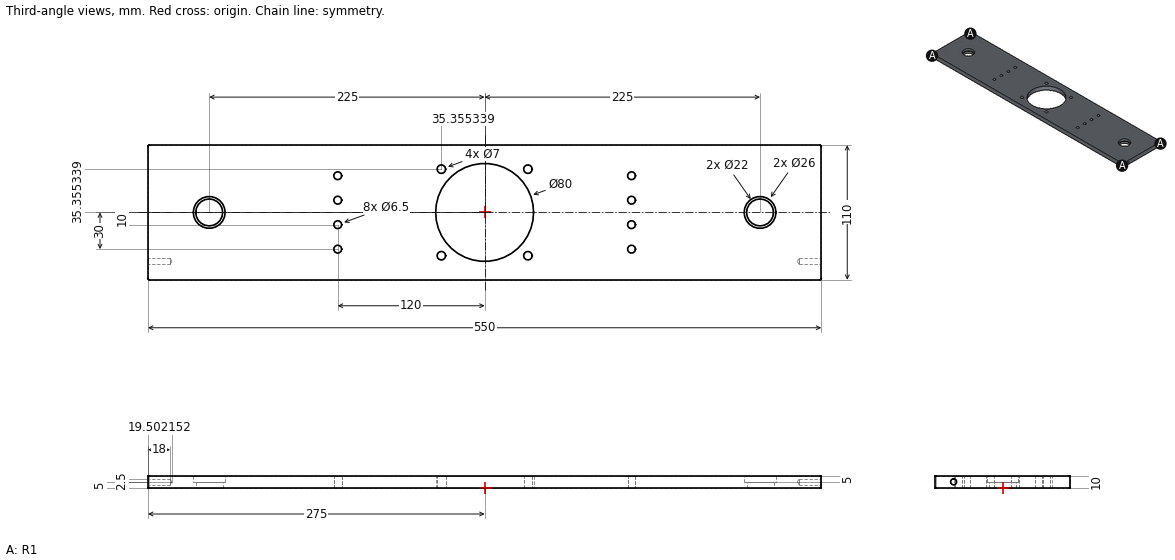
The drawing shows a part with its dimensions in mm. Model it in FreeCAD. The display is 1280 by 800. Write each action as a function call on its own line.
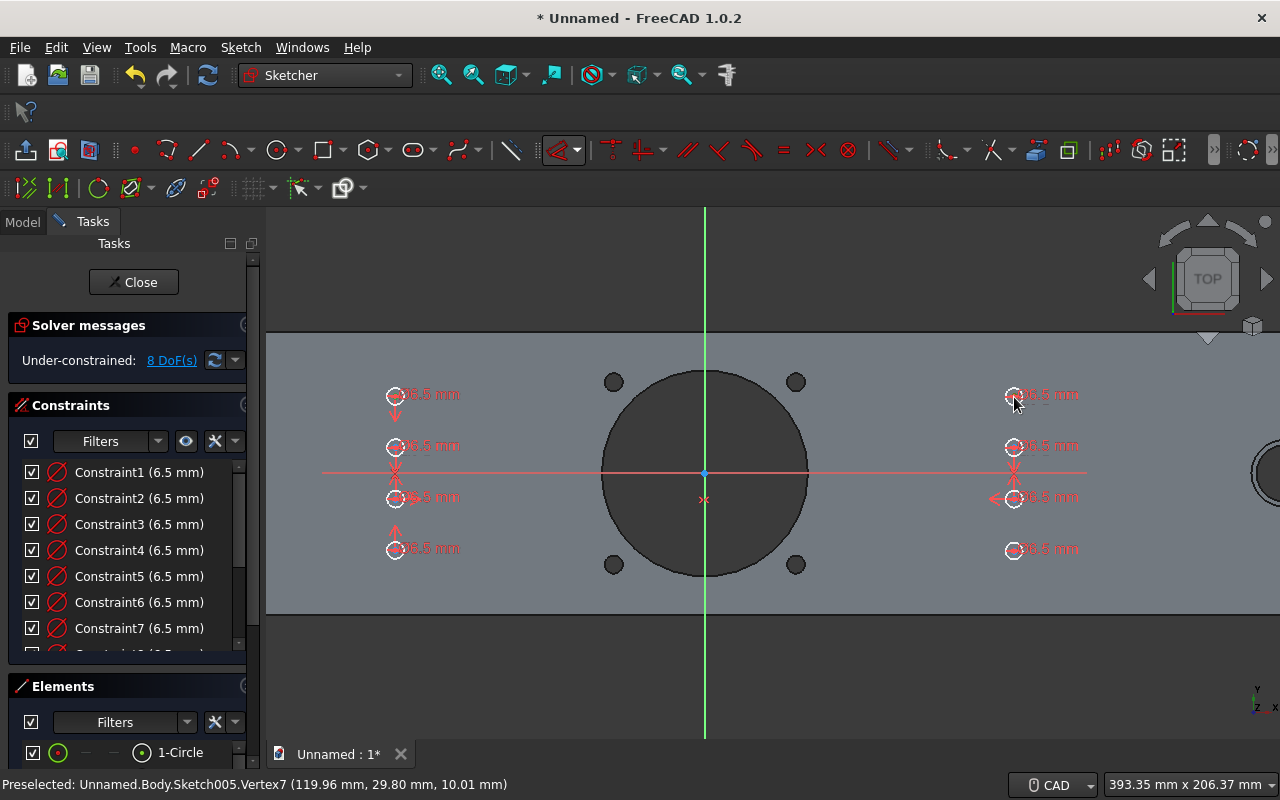
click(705, 677)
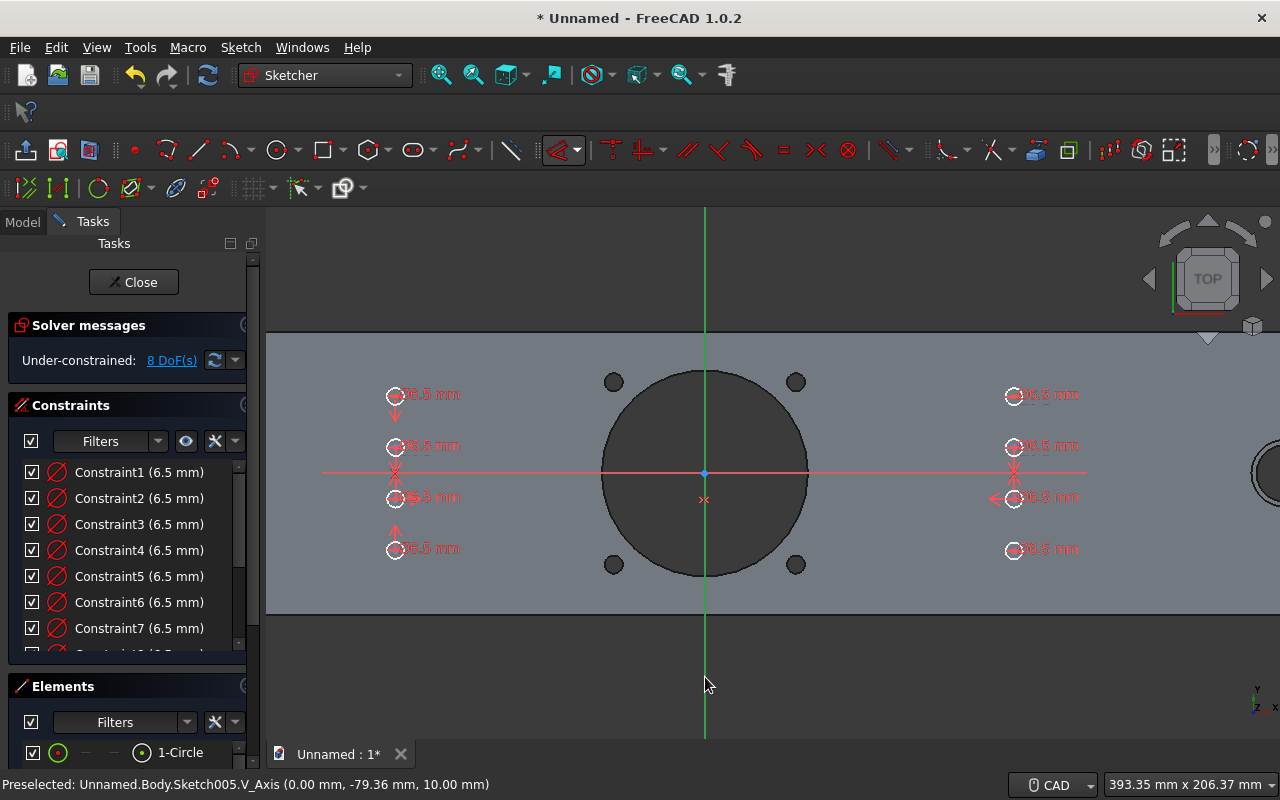
key(s)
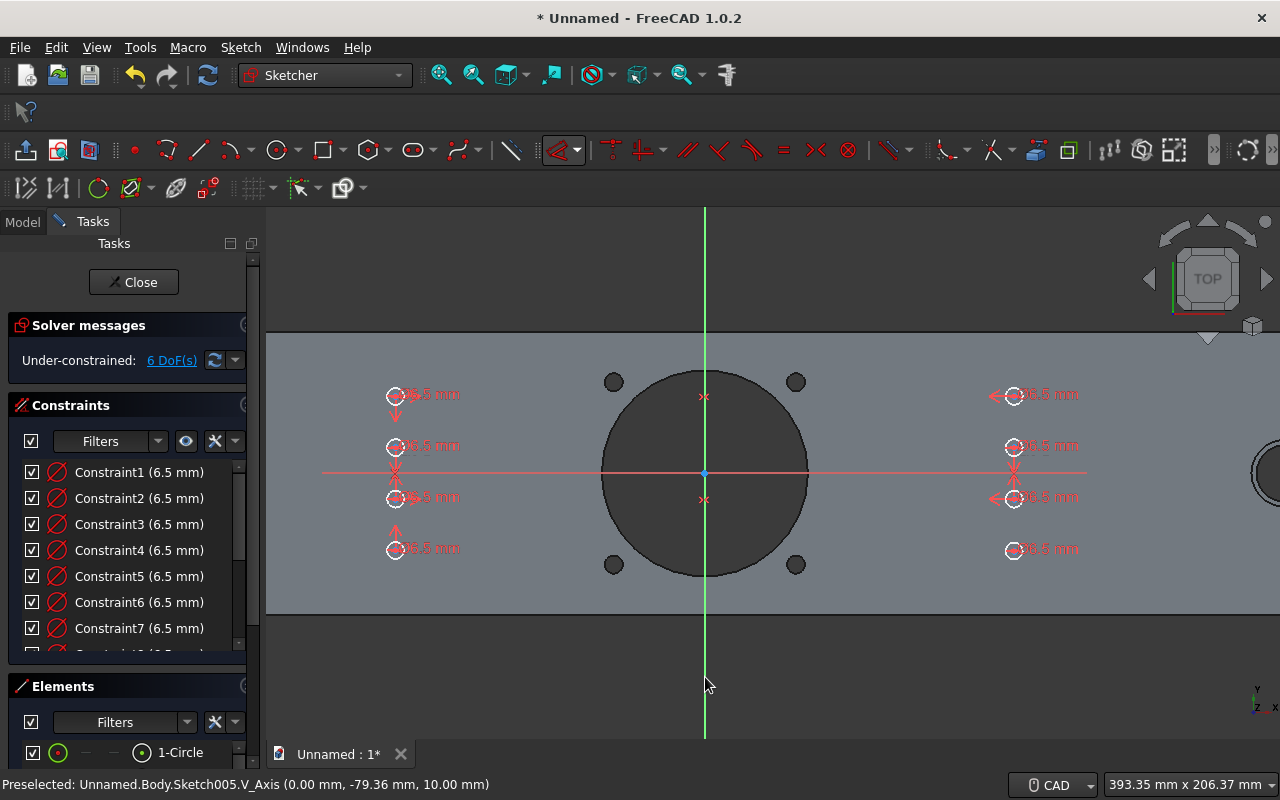
click(396, 550)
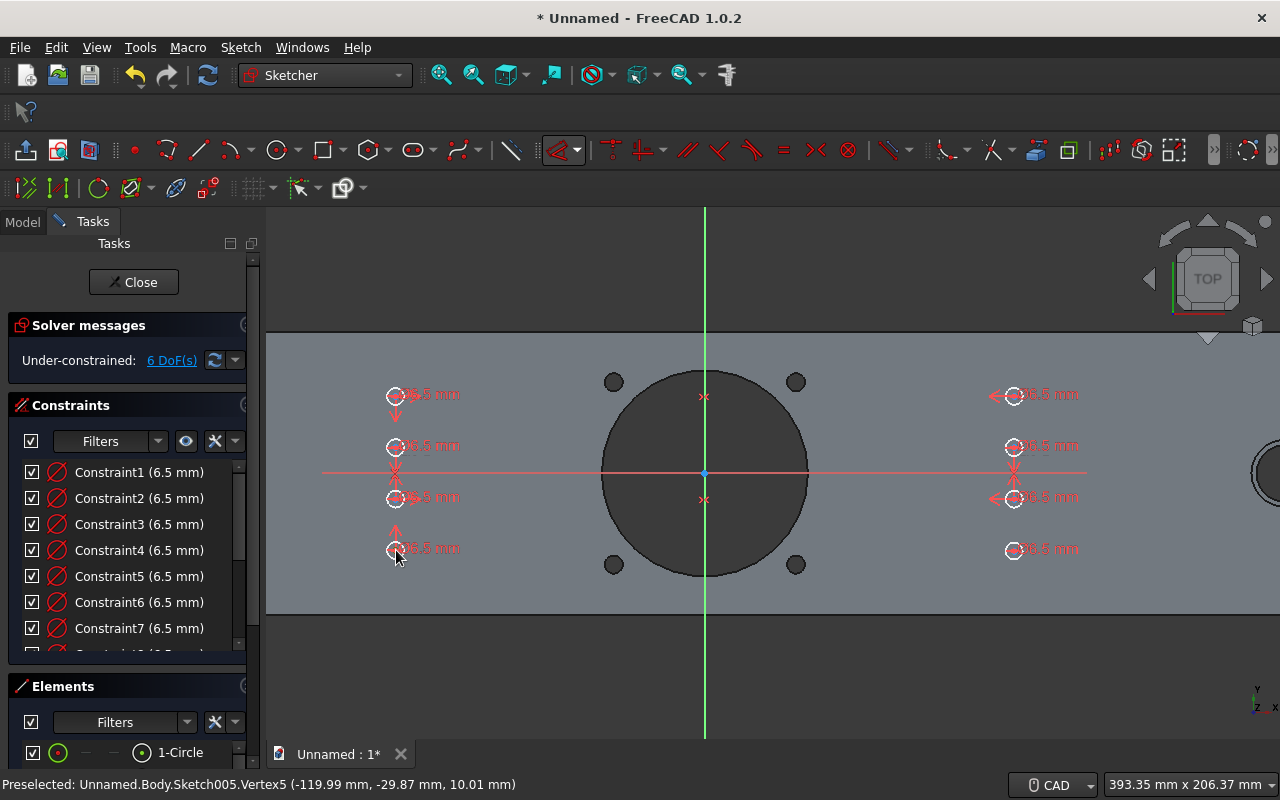
click(1014, 551)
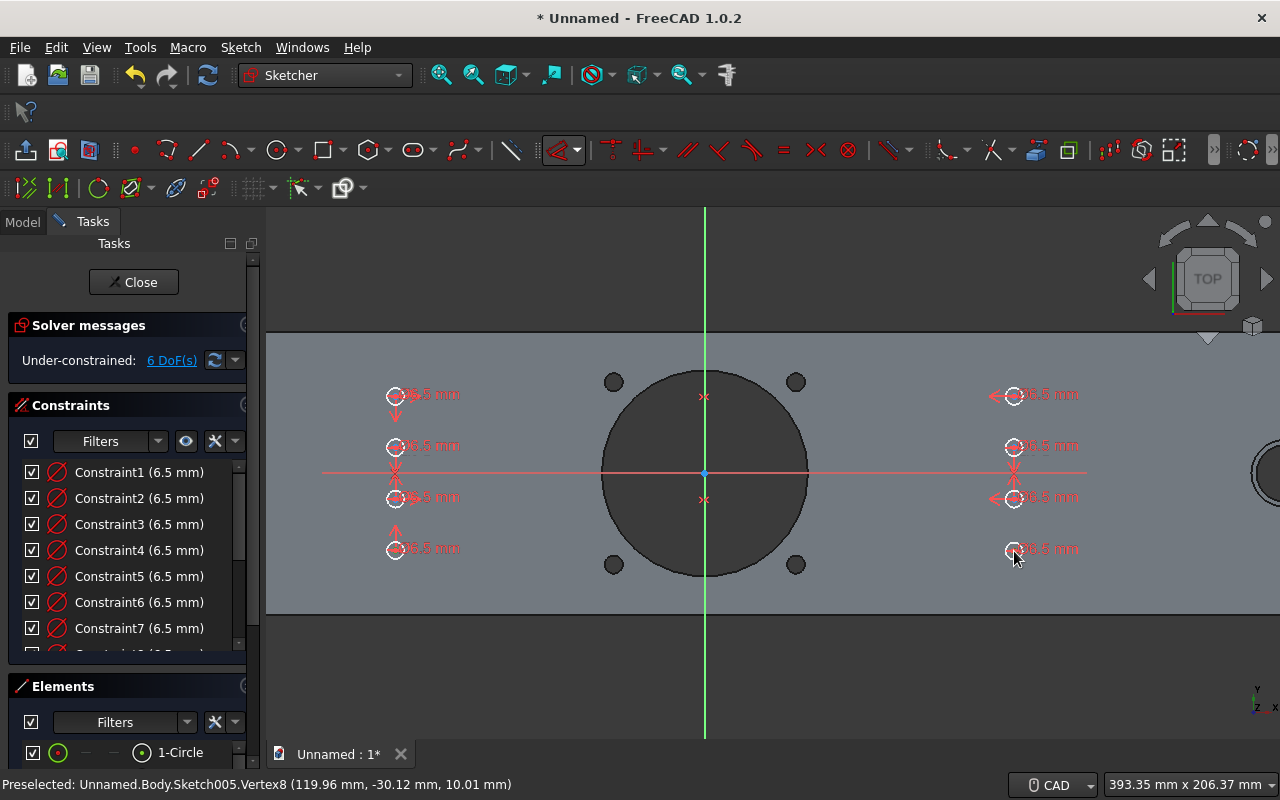
click(705, 677)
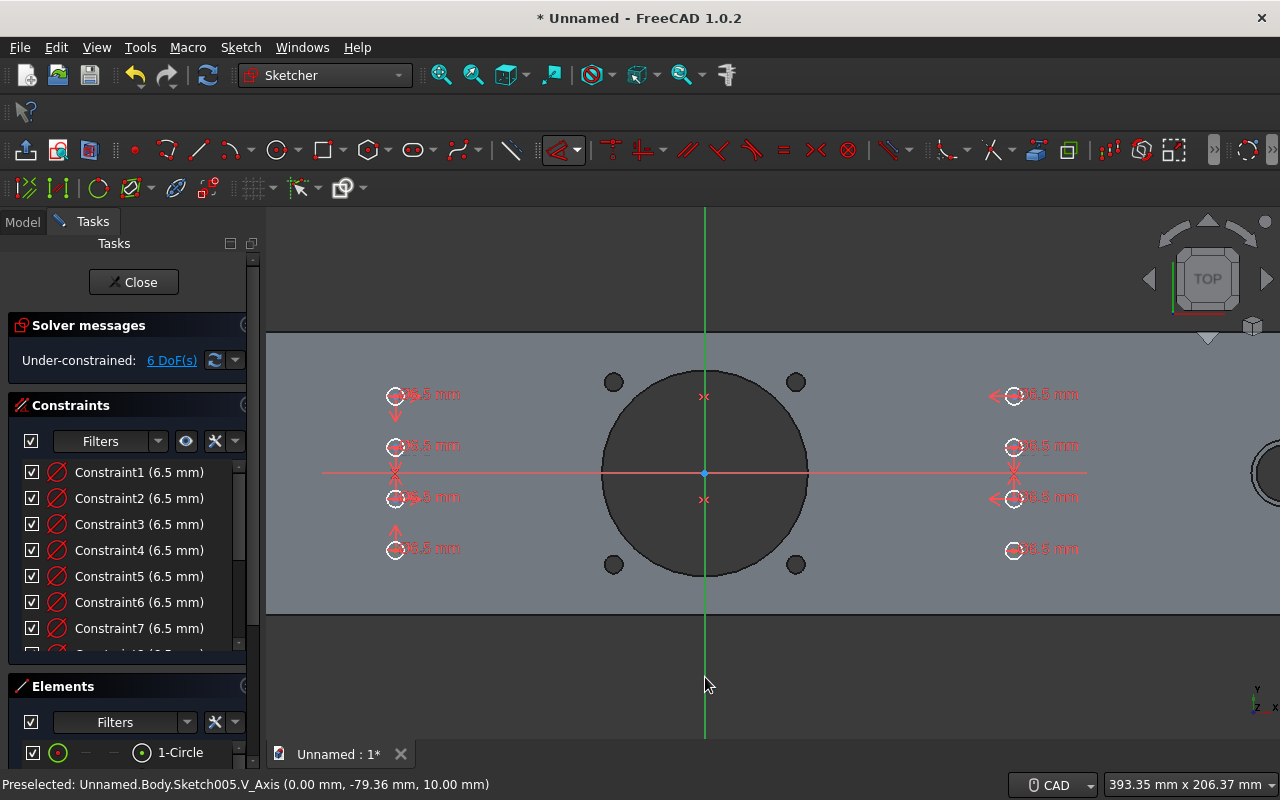
key(s)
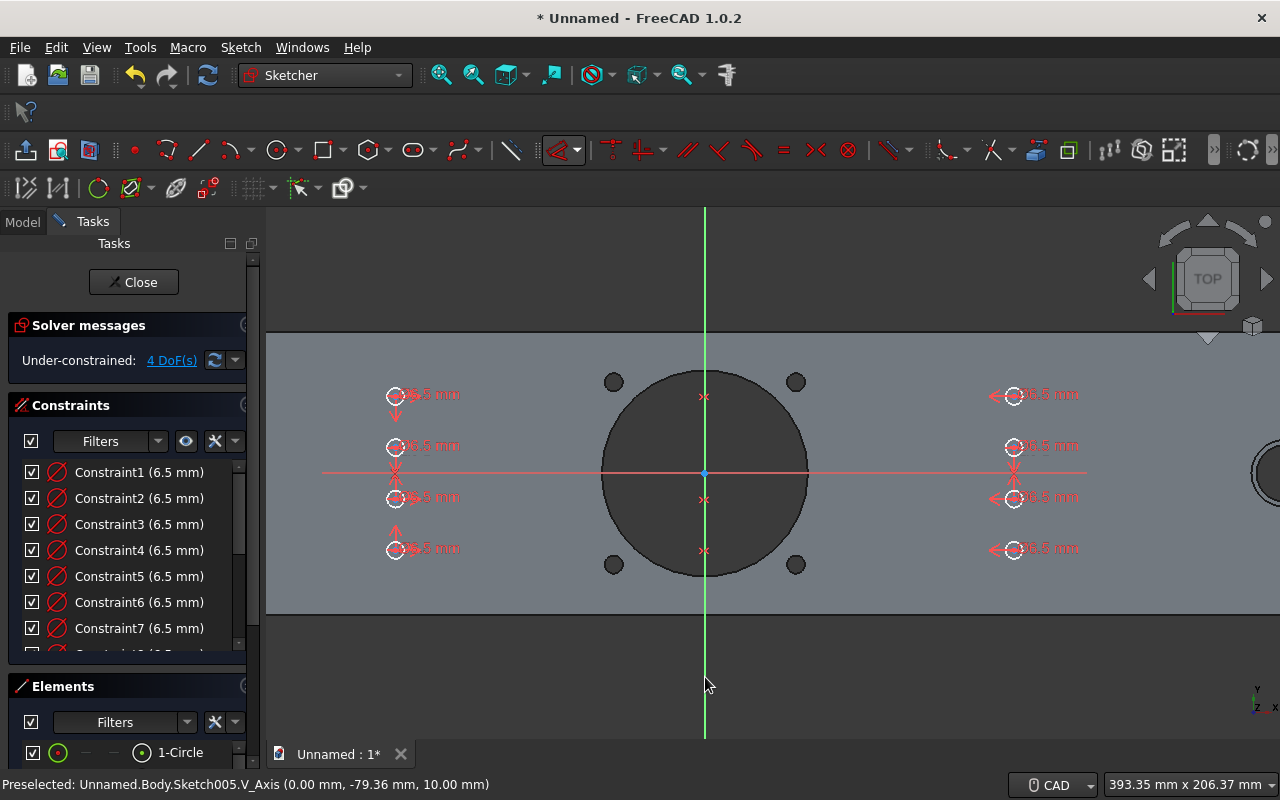
scroll(396, 499, up, 3)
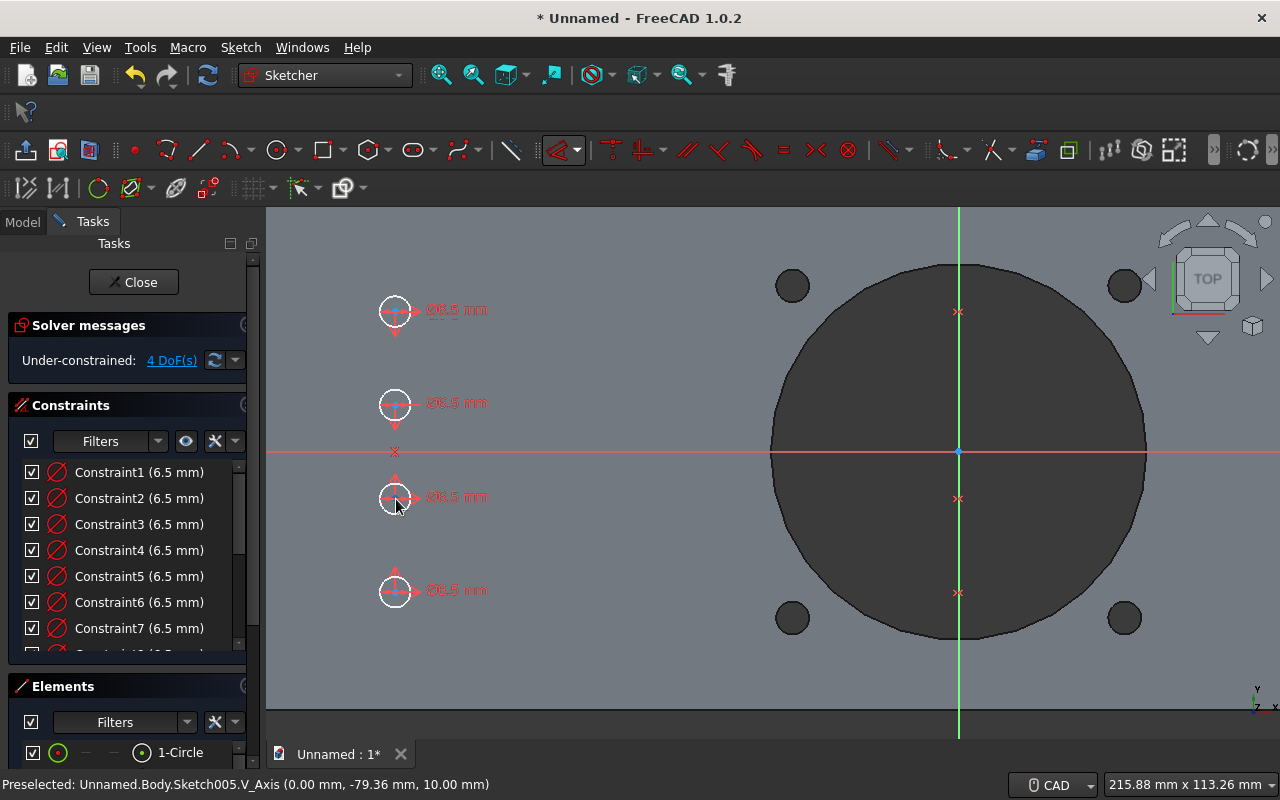
click(395, 499)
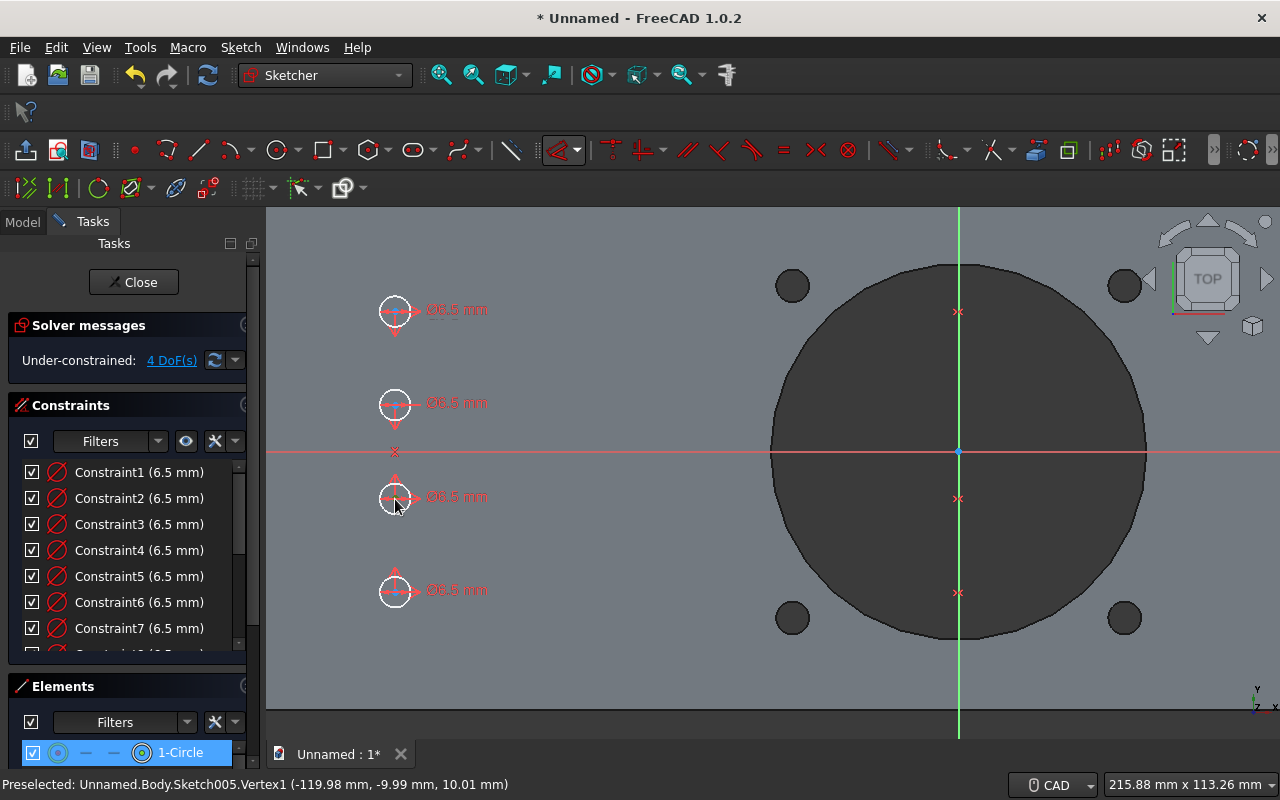
key(i)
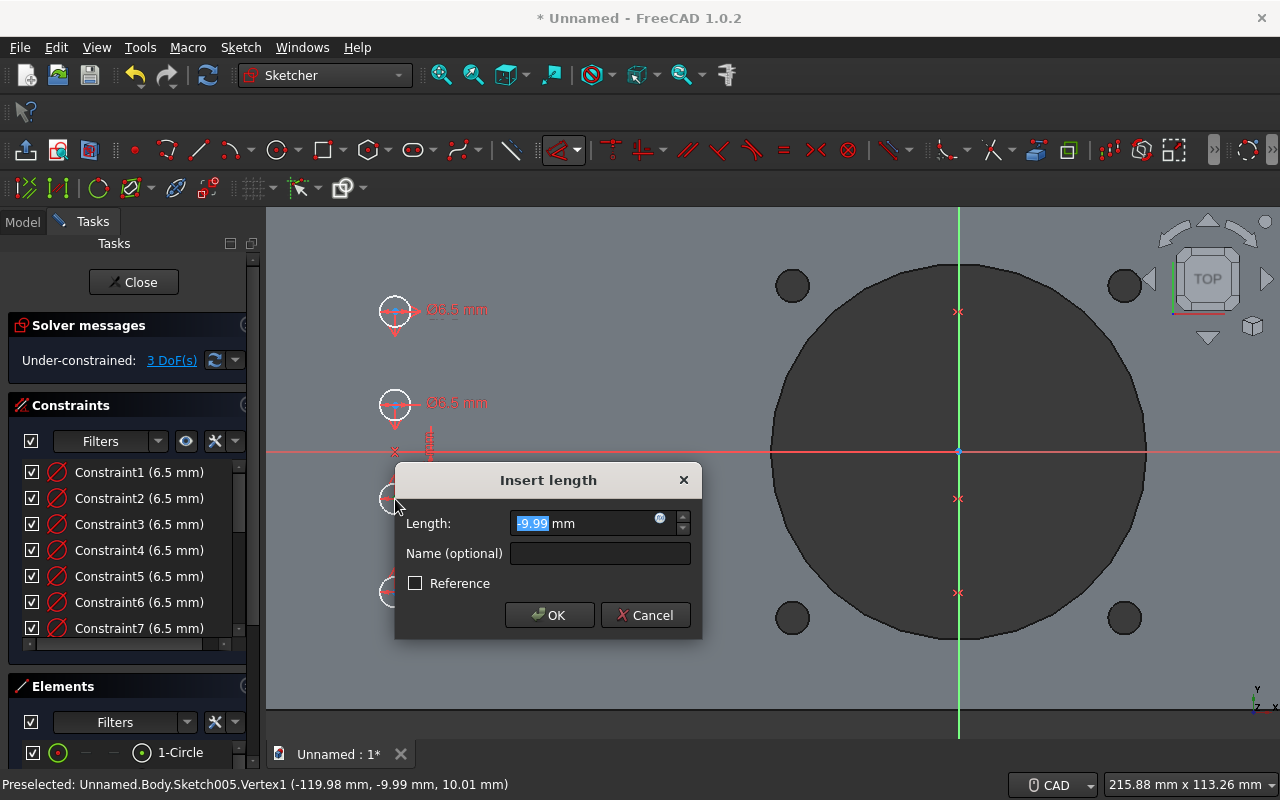
text(-10)
key(Return)